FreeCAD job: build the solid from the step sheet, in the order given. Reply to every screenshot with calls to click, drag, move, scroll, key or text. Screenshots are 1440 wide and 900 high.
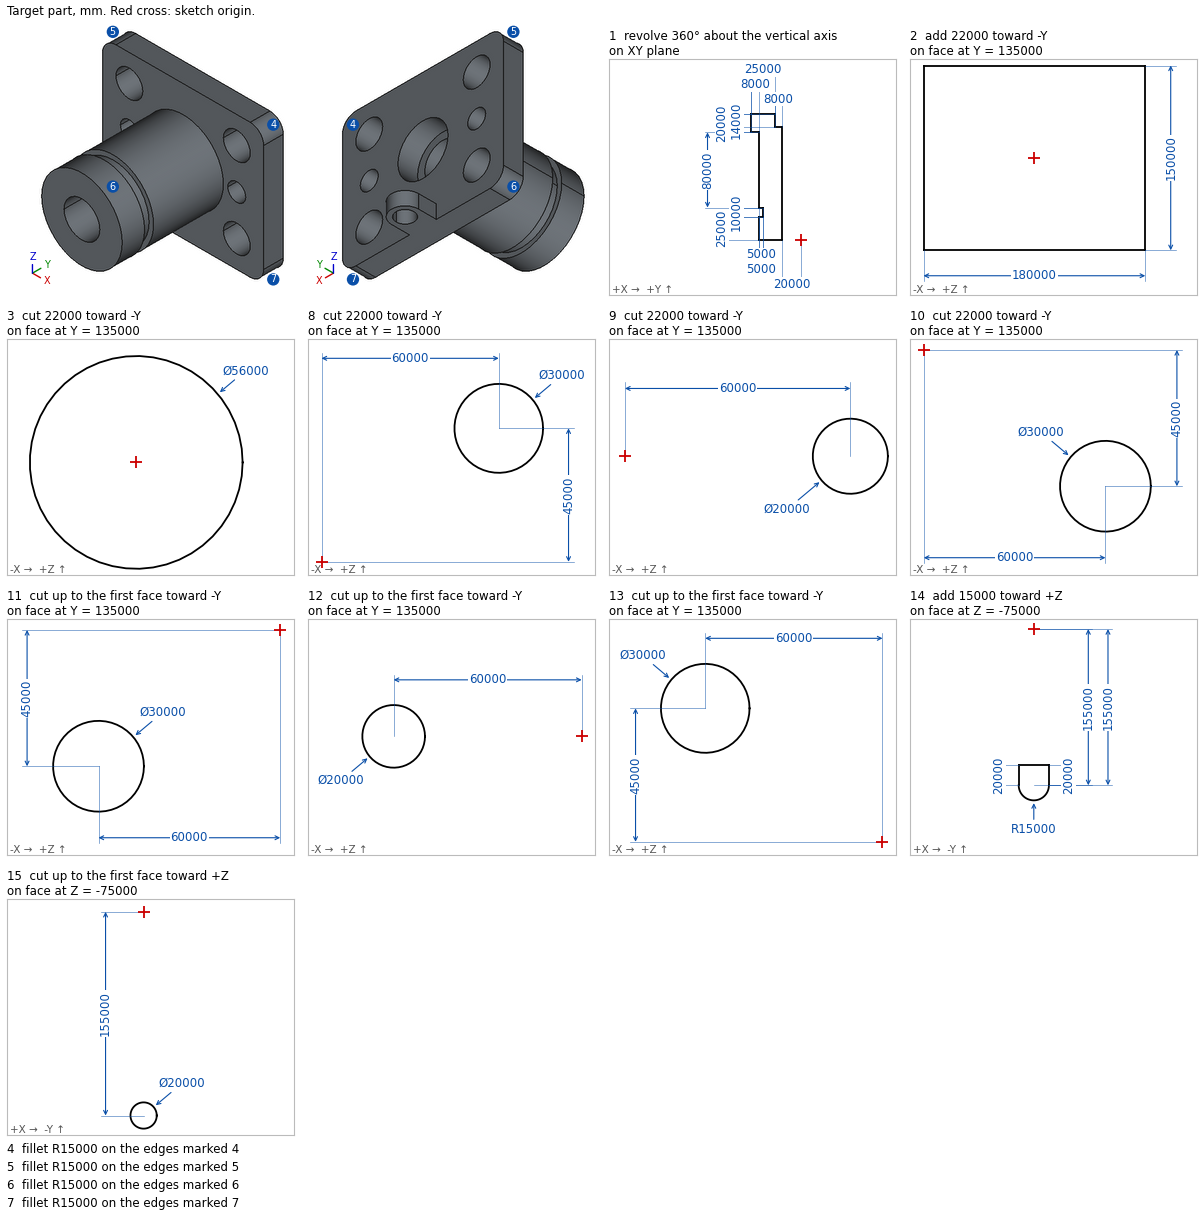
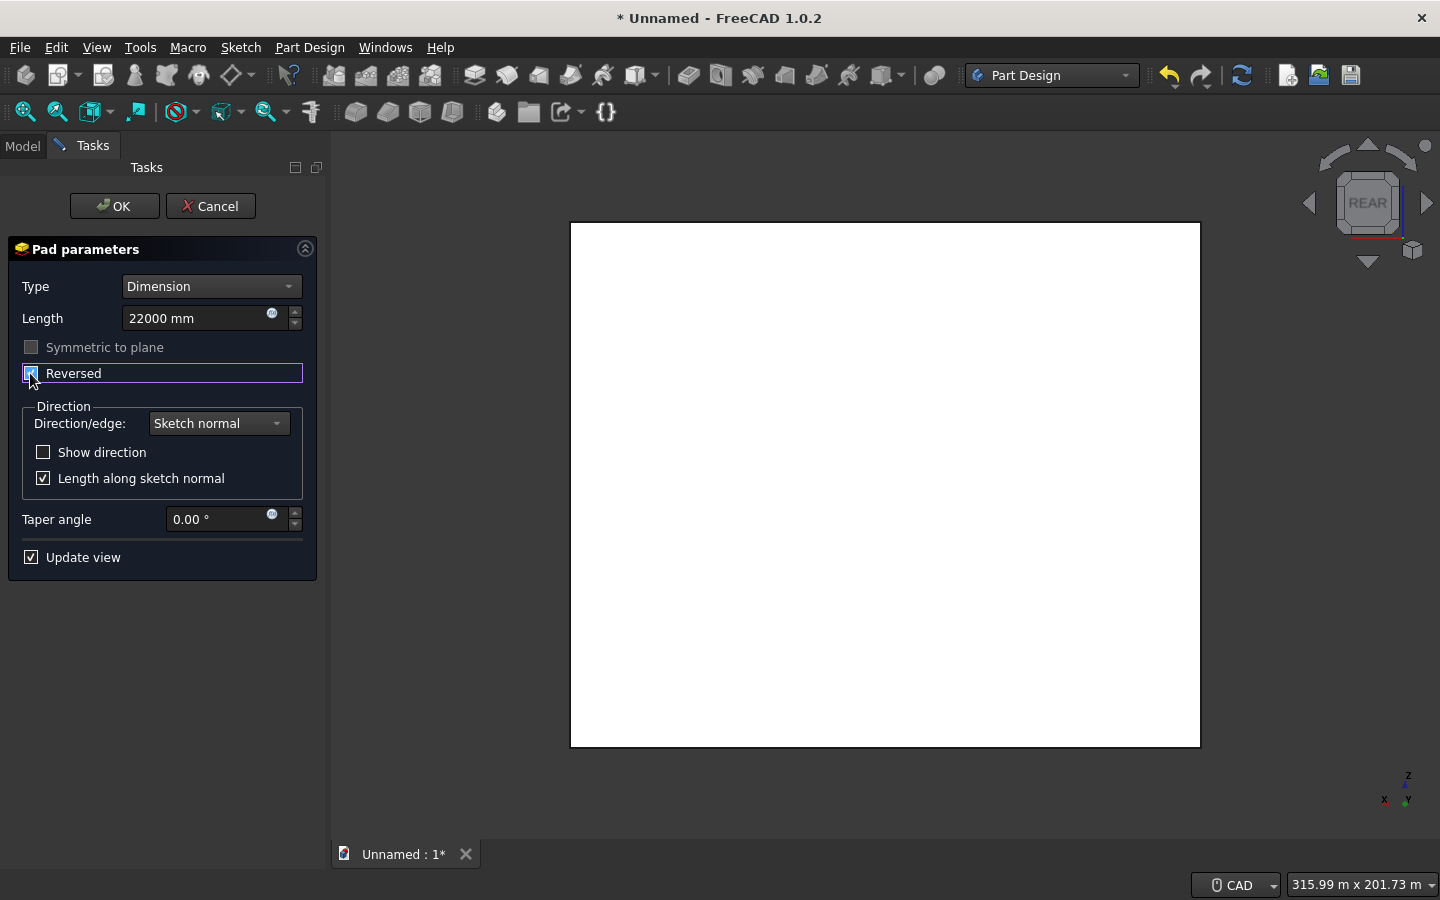
click(115, 206)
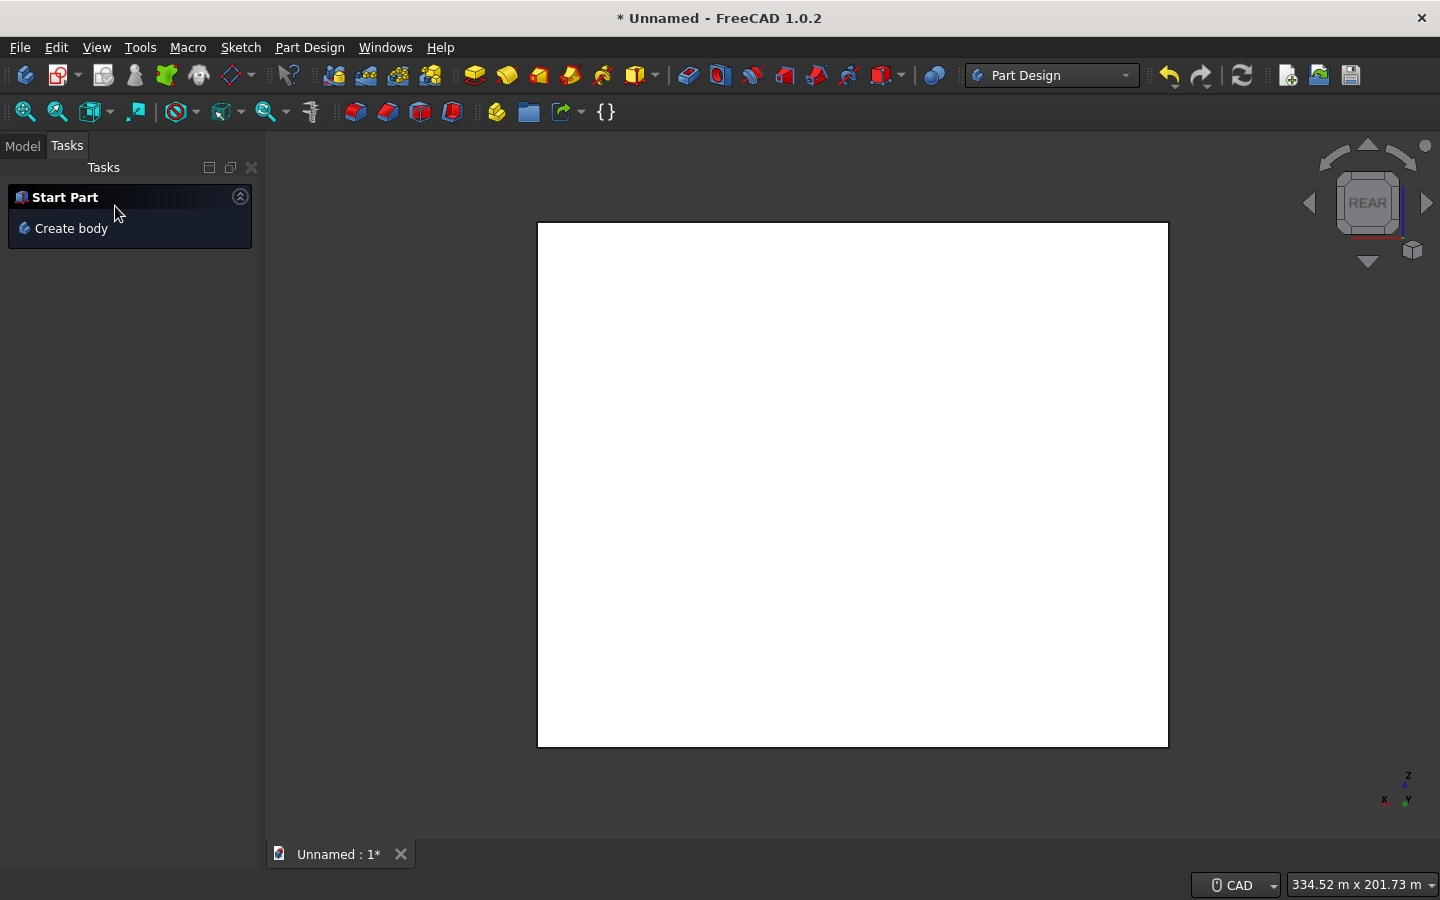
click(853, 484)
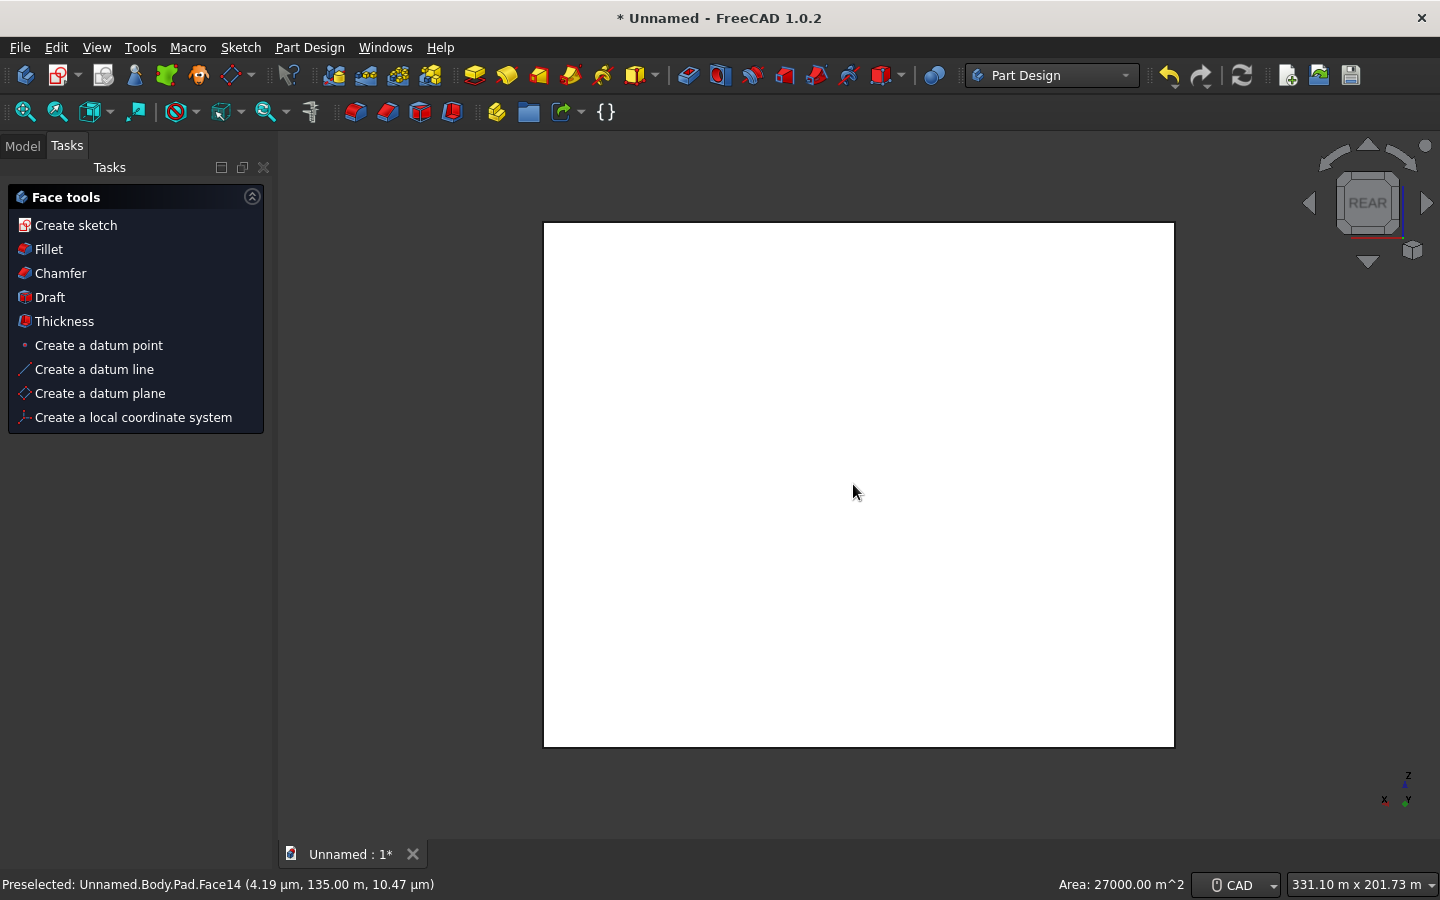
click(58, 76)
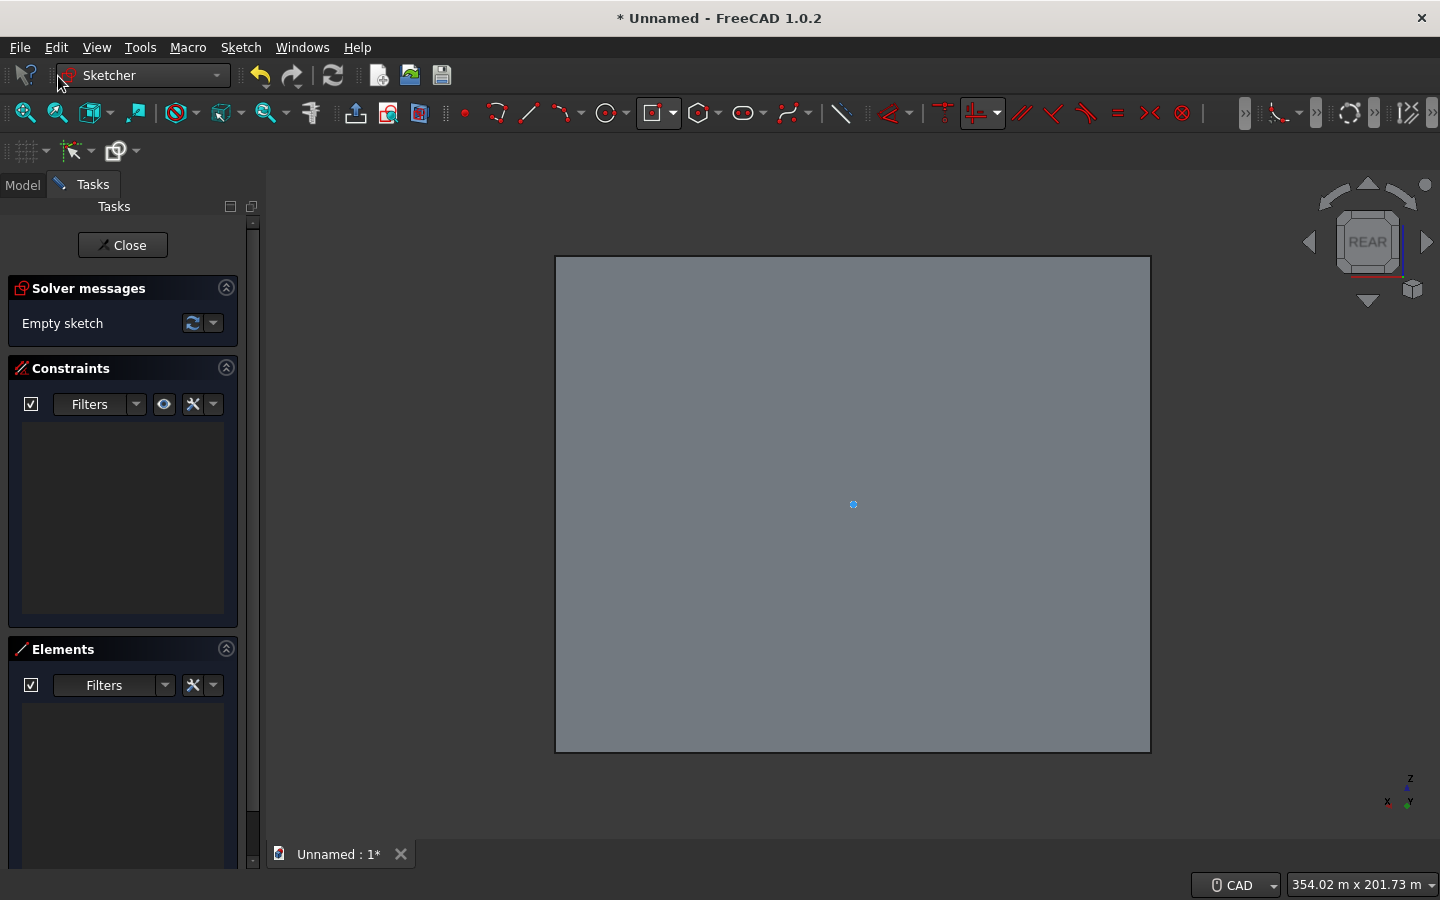
scroll(909, 505, up, 4)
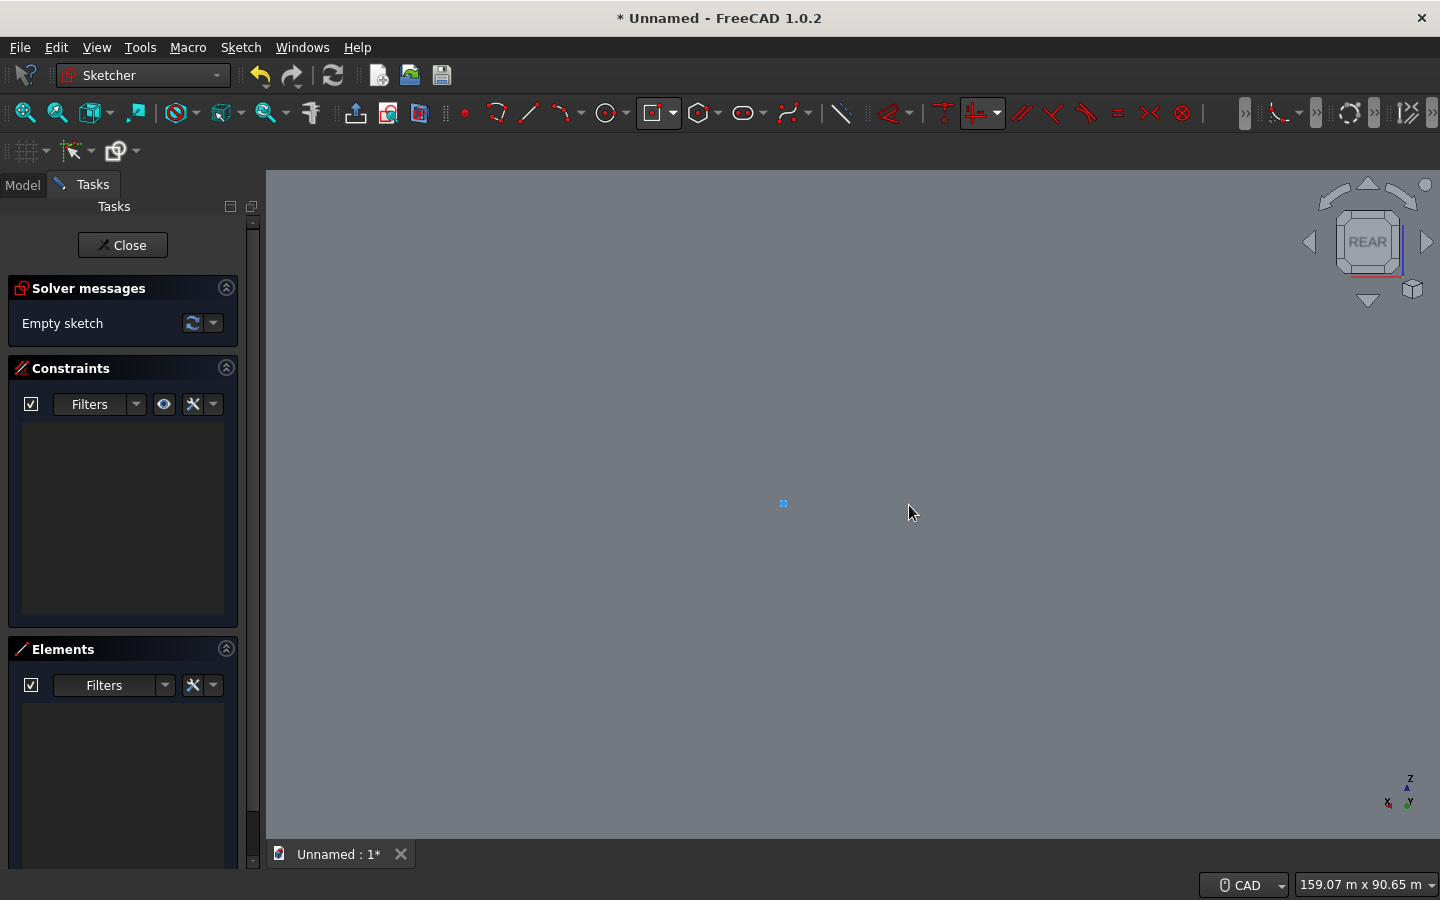
click(606, 114)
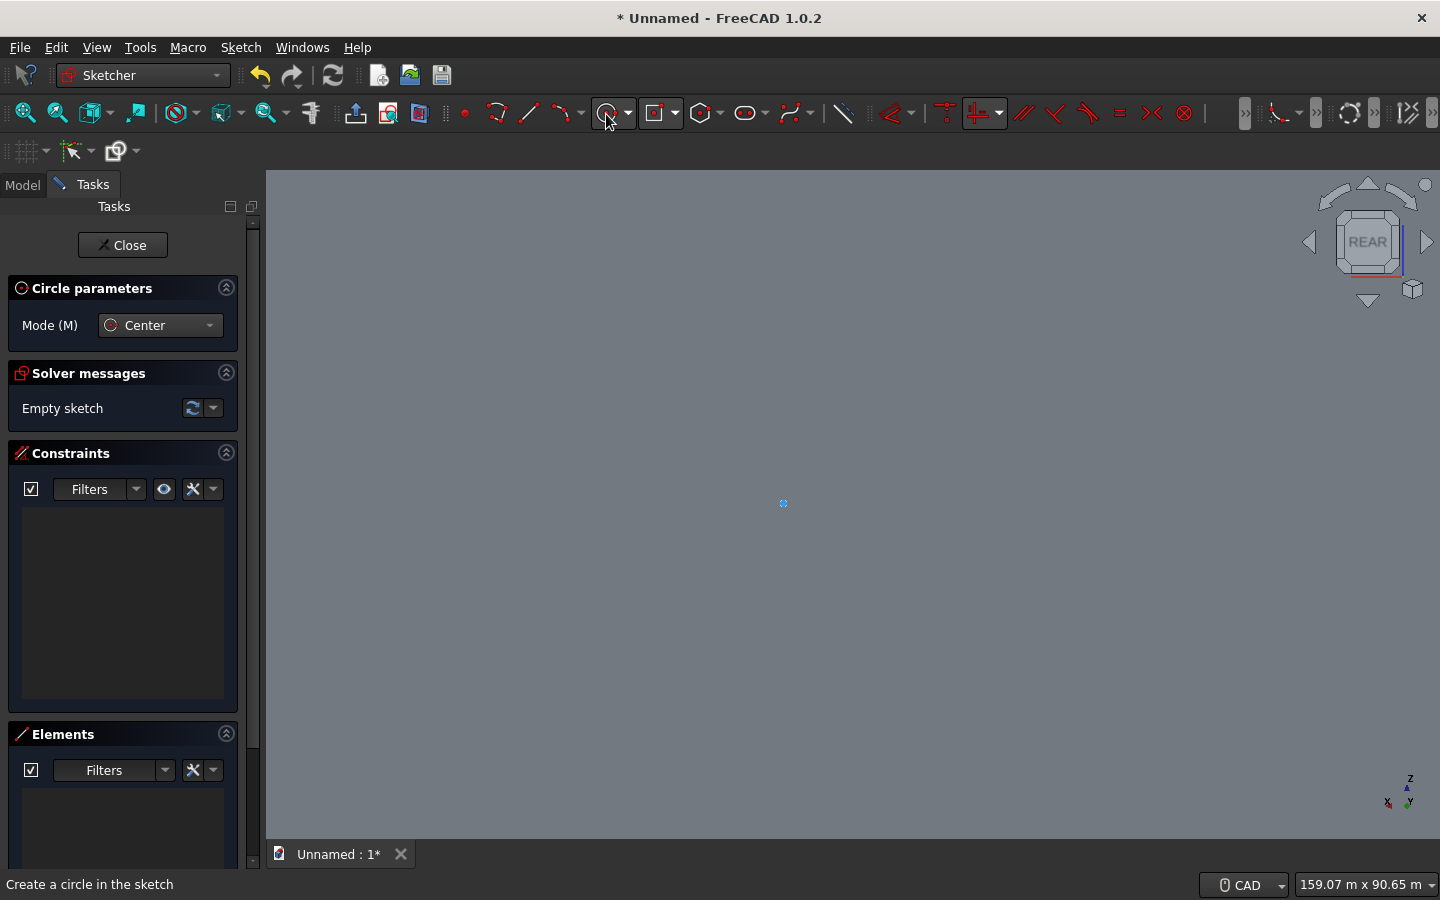
click(784, 503)
click(930, 357)
key(Escape)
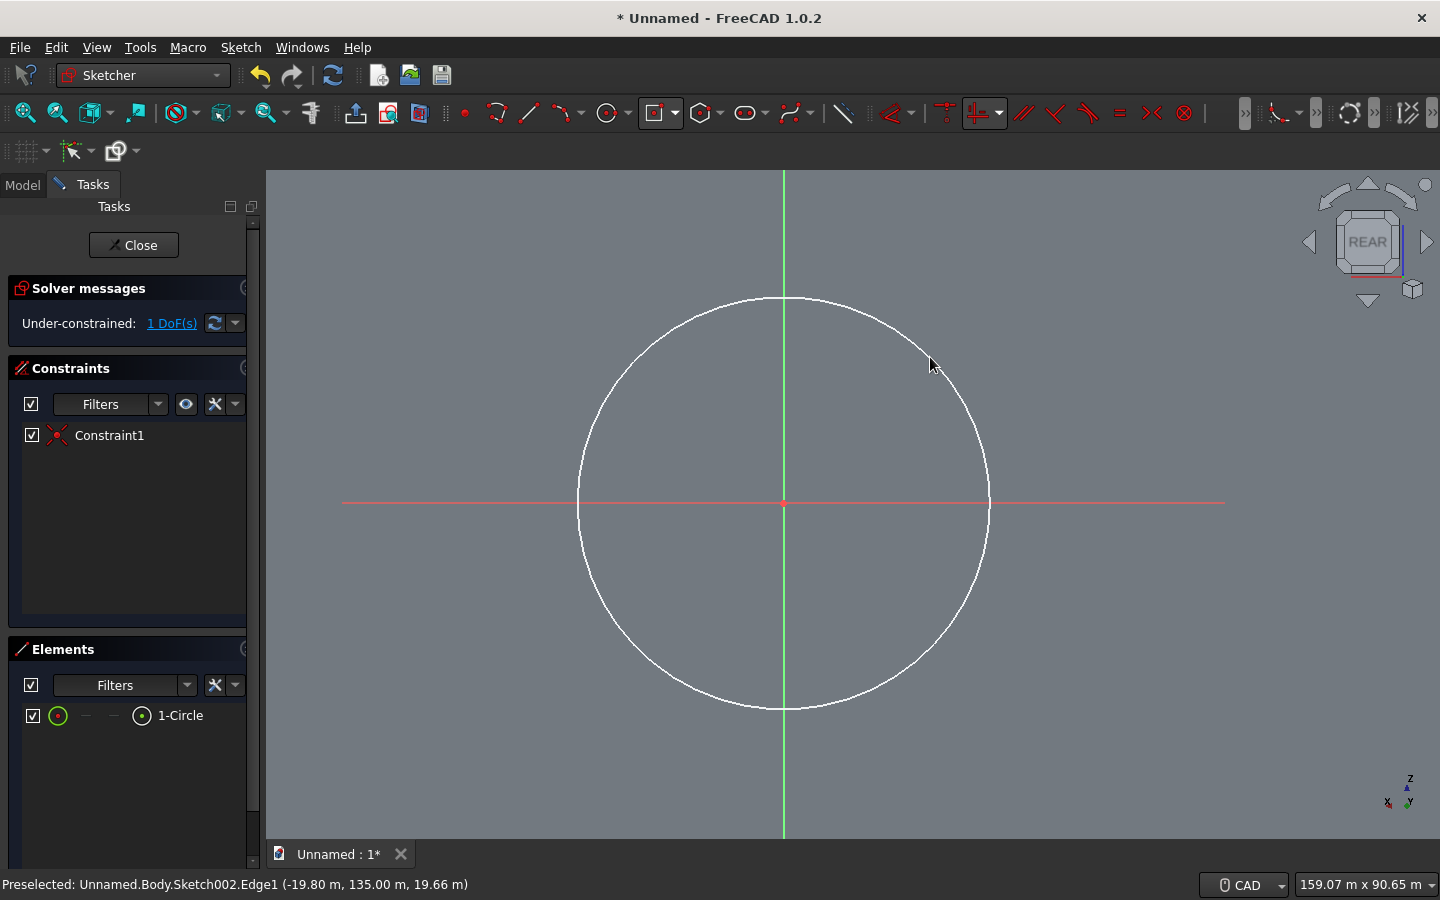
click(890, 114)